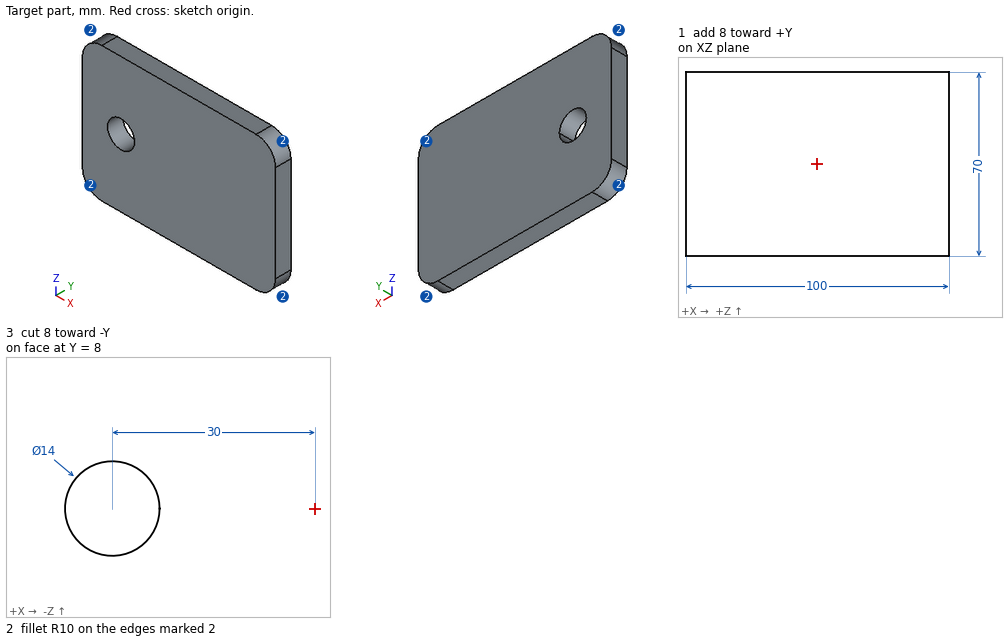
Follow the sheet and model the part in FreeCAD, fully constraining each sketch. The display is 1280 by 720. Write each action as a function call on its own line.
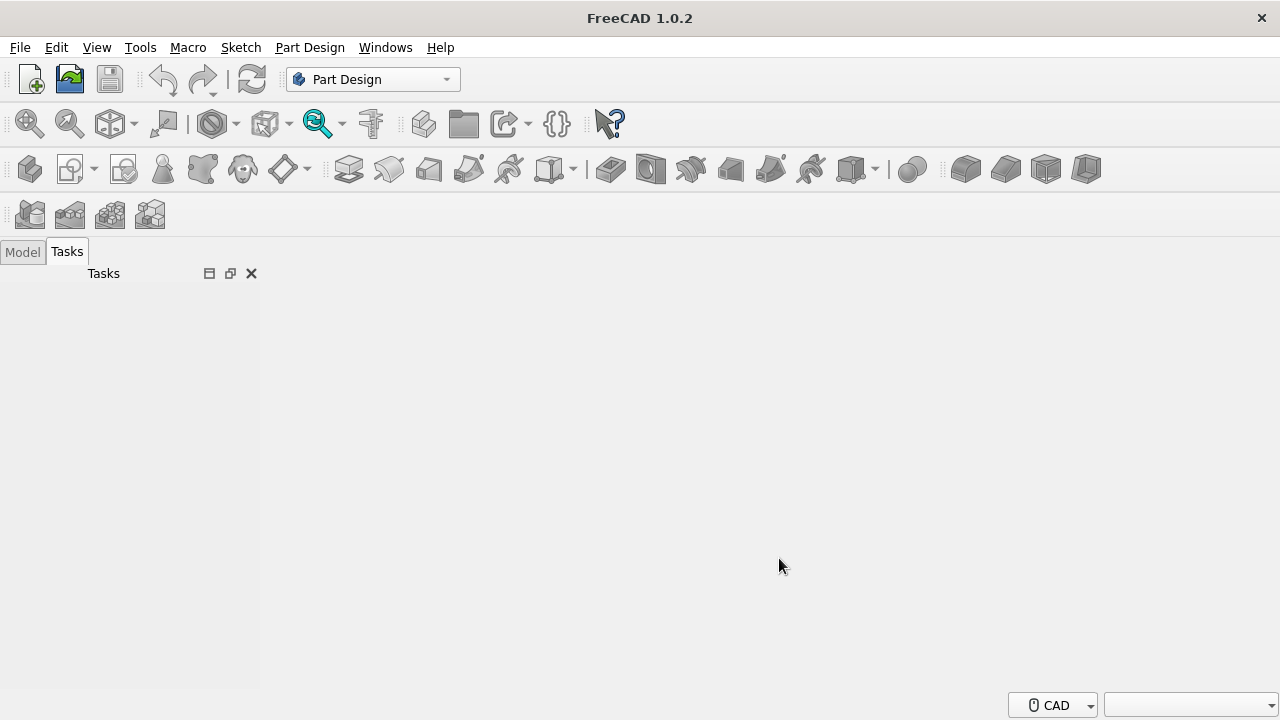
click(30, 80)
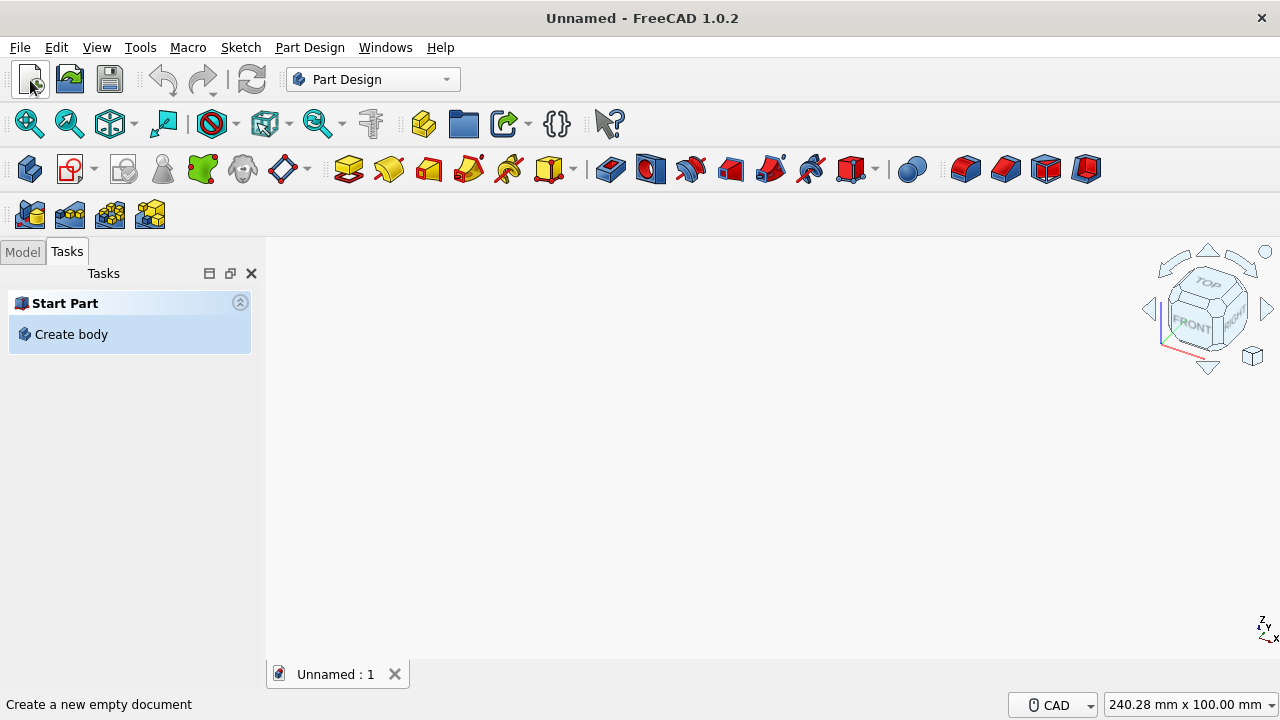
click(70, 170)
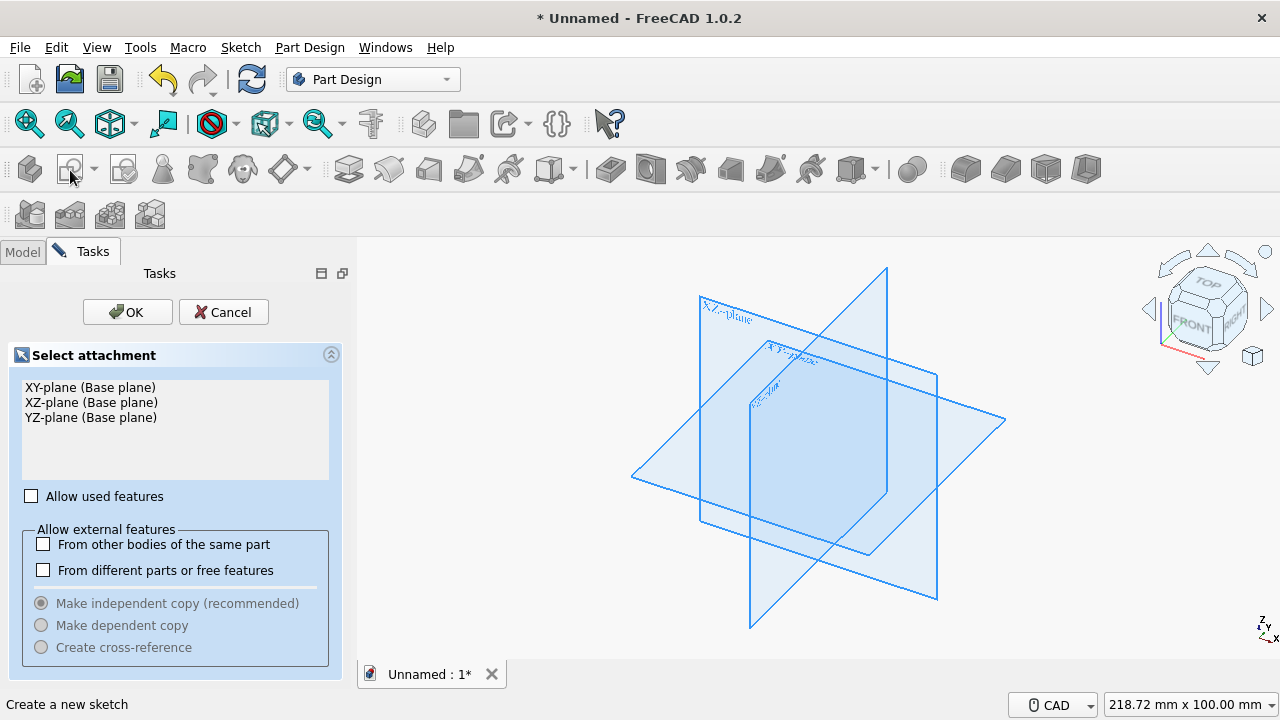
click(82, 402)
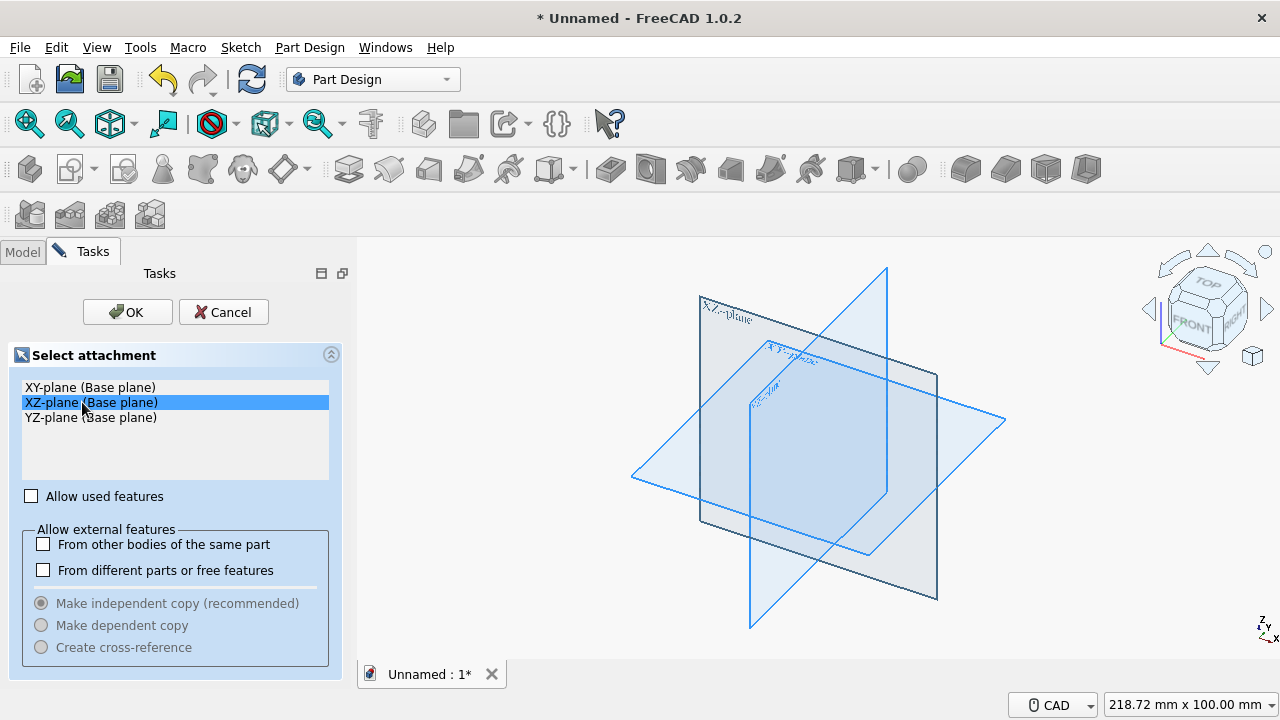
click(128, 312)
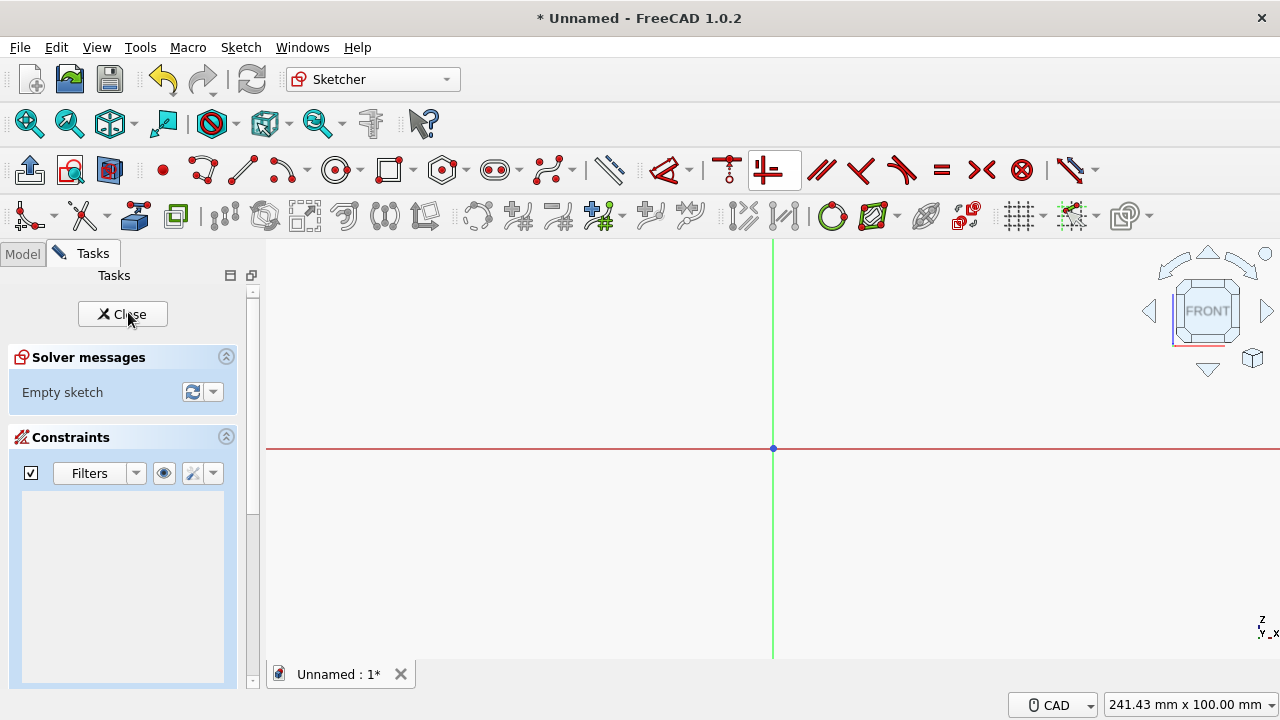
click(416, 170)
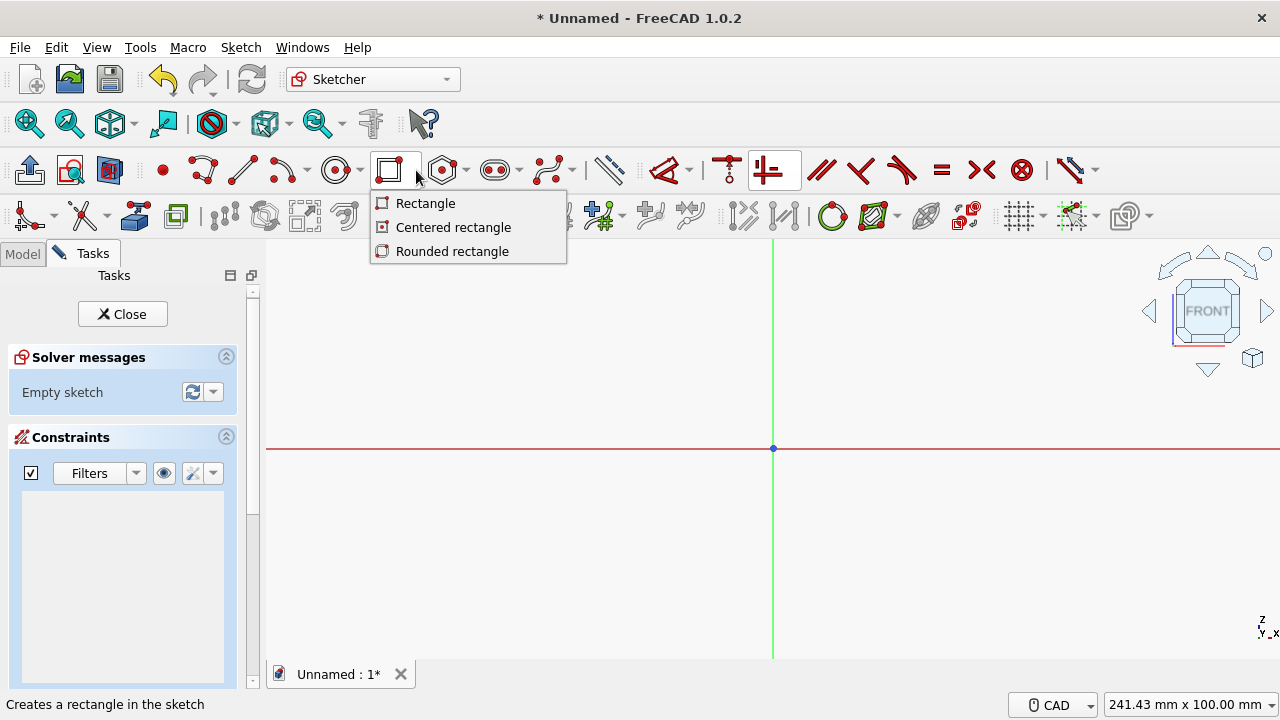
click(468, 227)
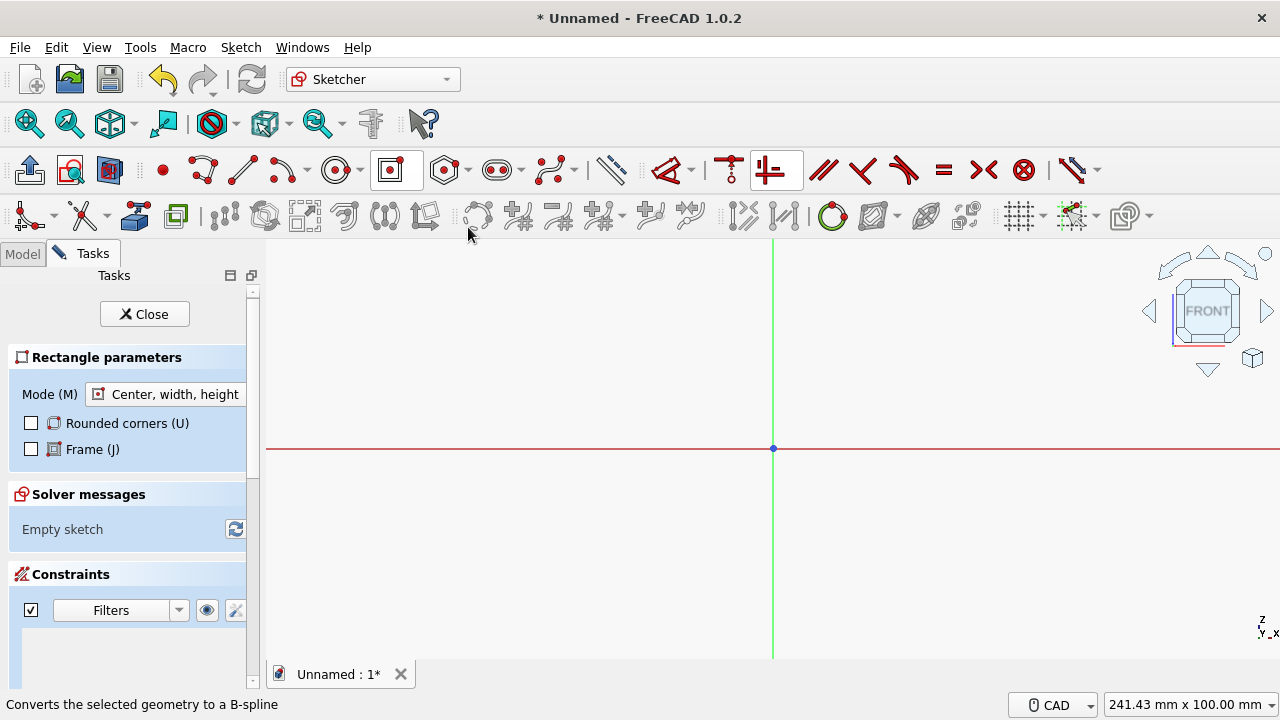
click(773, 449)
click(983, 302)
key(Escape)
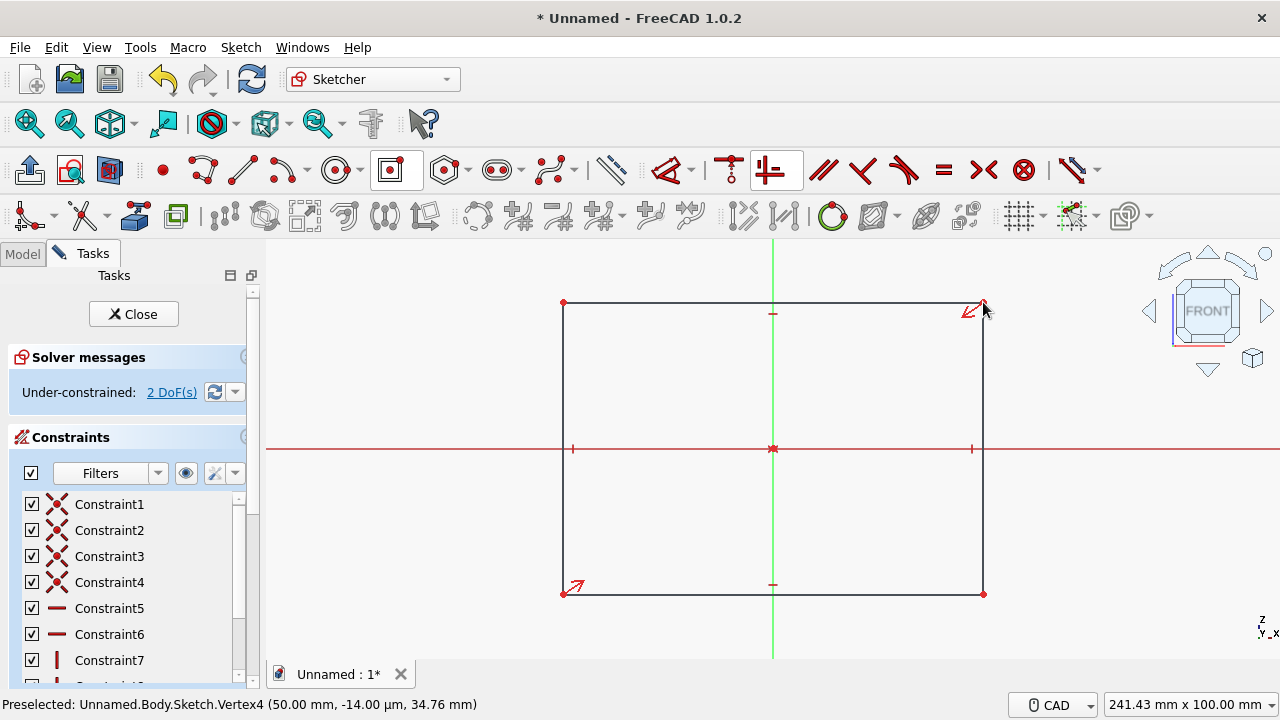
click(983, 507)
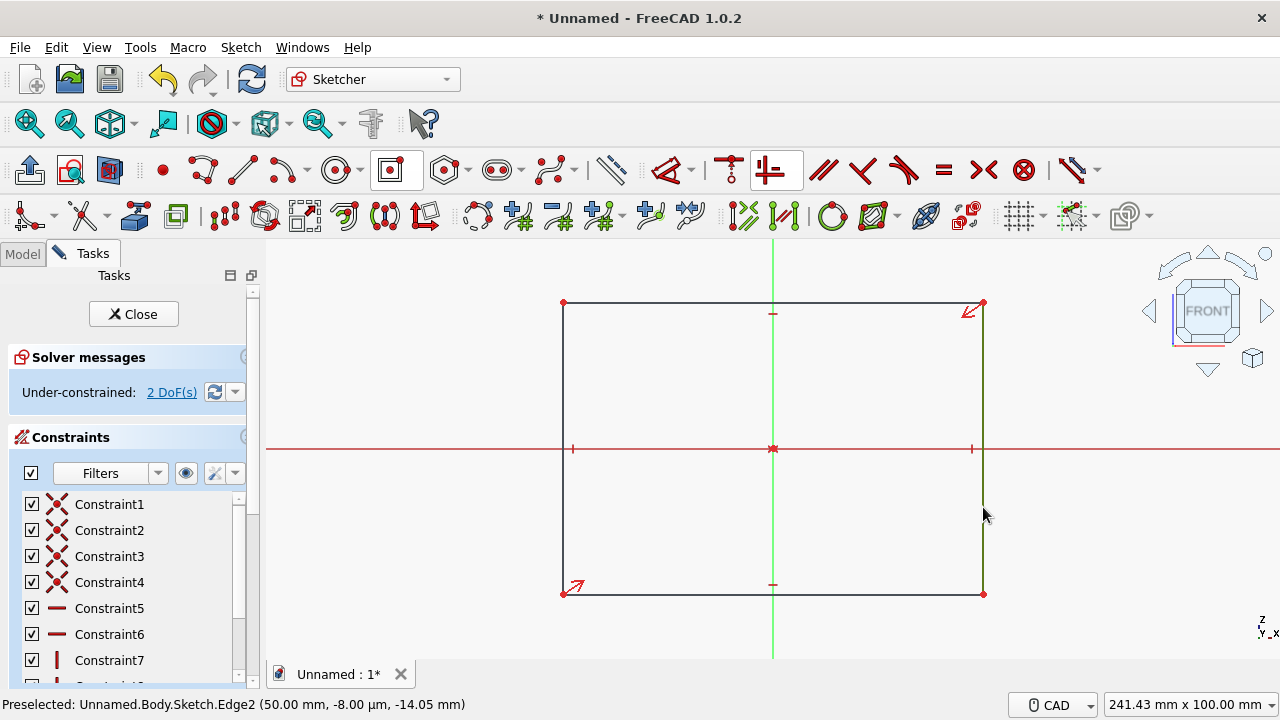
click(694, 170)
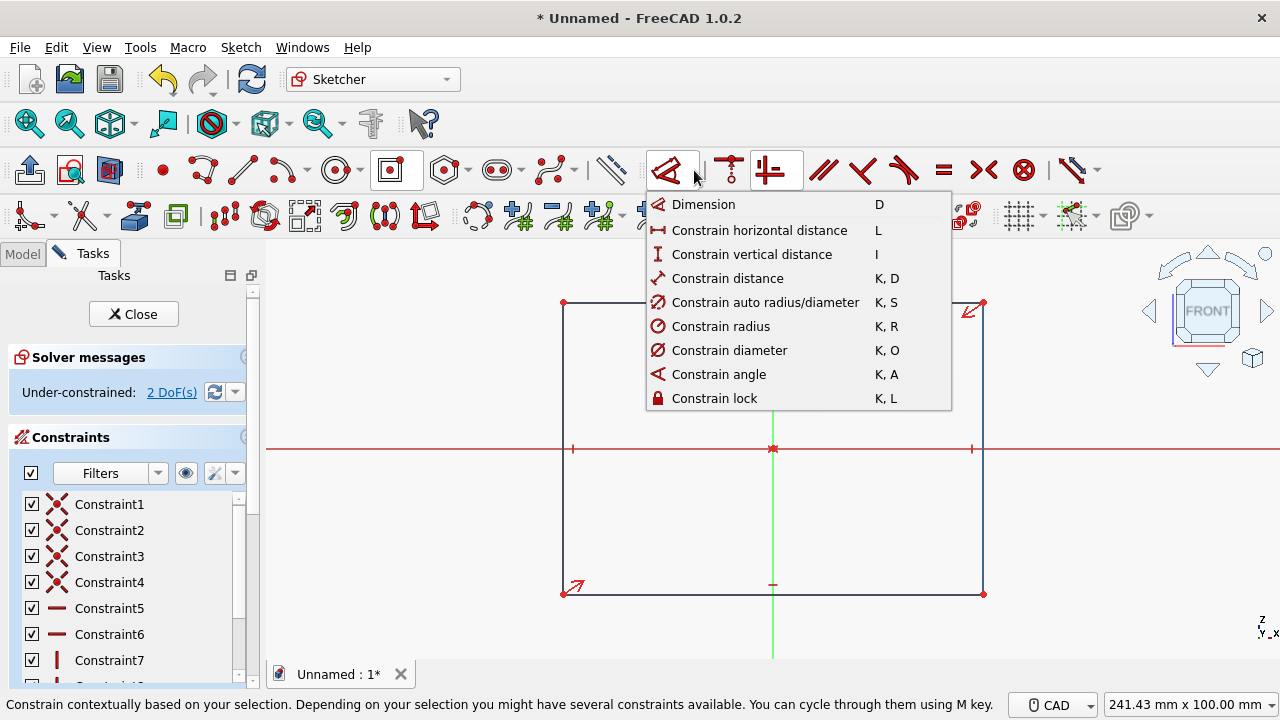
click(799, 254)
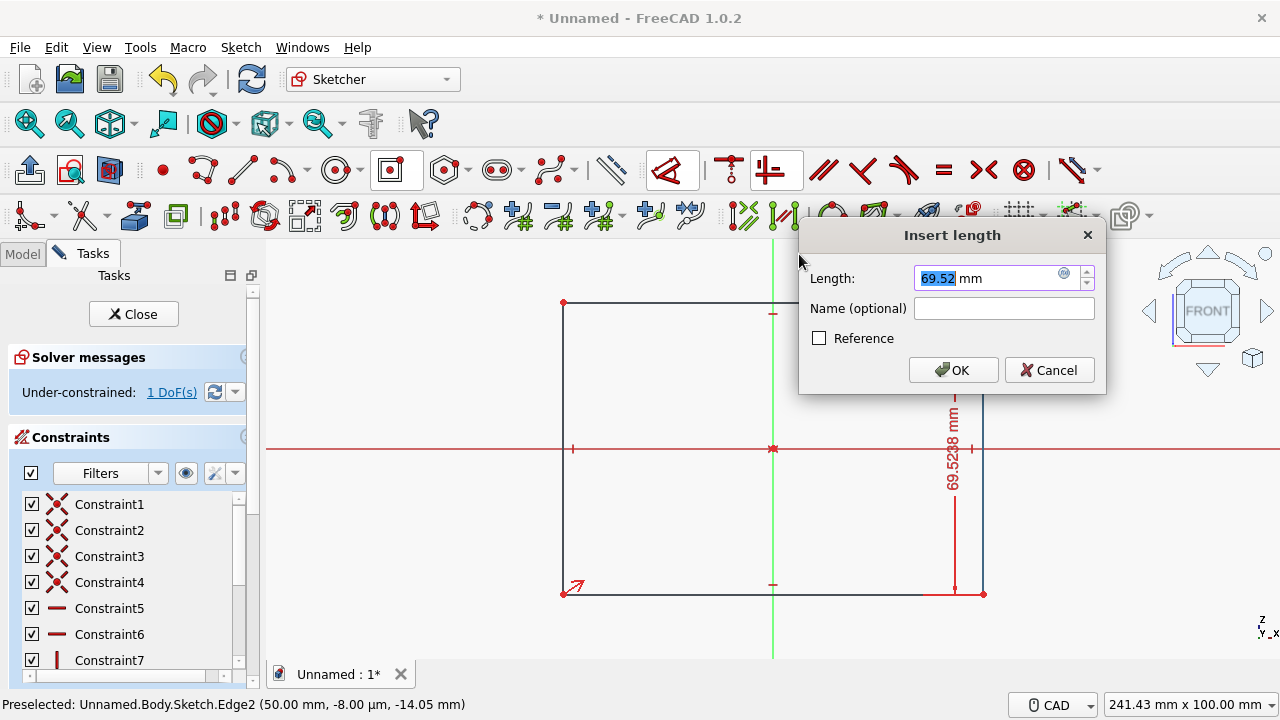
text(70)
key(Return)